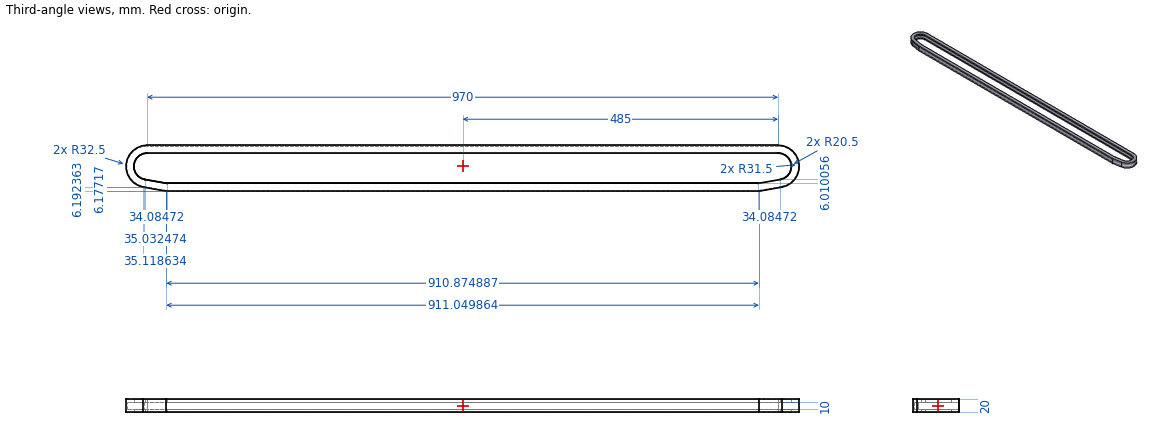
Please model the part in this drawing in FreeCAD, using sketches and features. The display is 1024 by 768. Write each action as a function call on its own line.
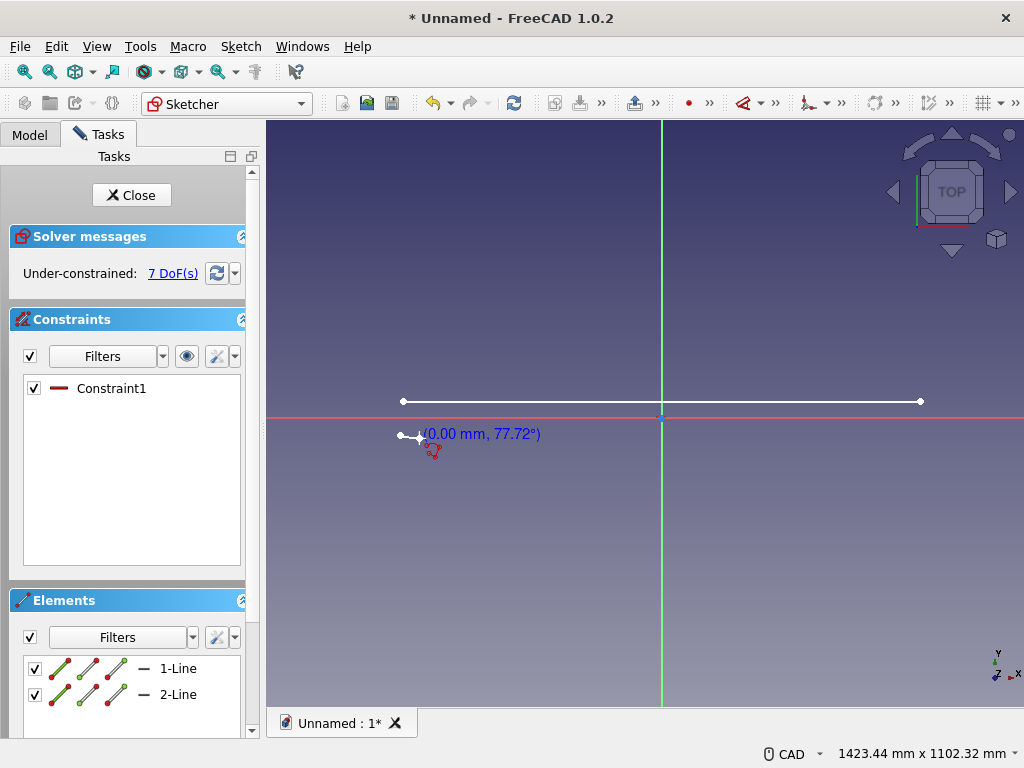
scroll(403, 401, down, 2)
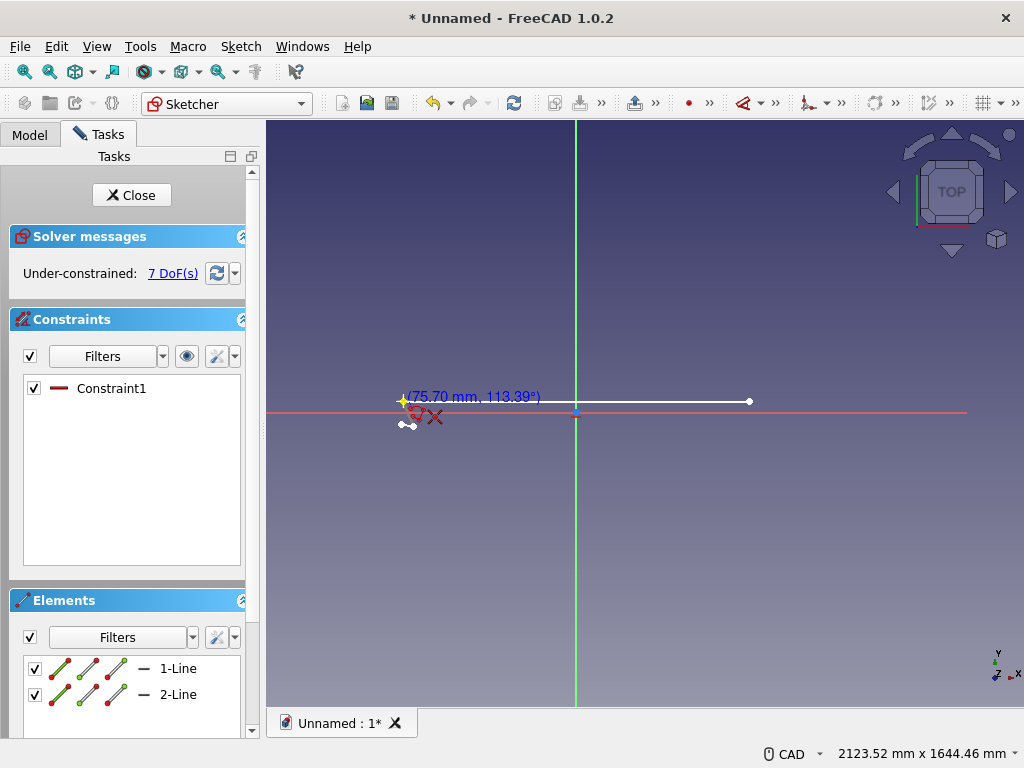
click(739, 426)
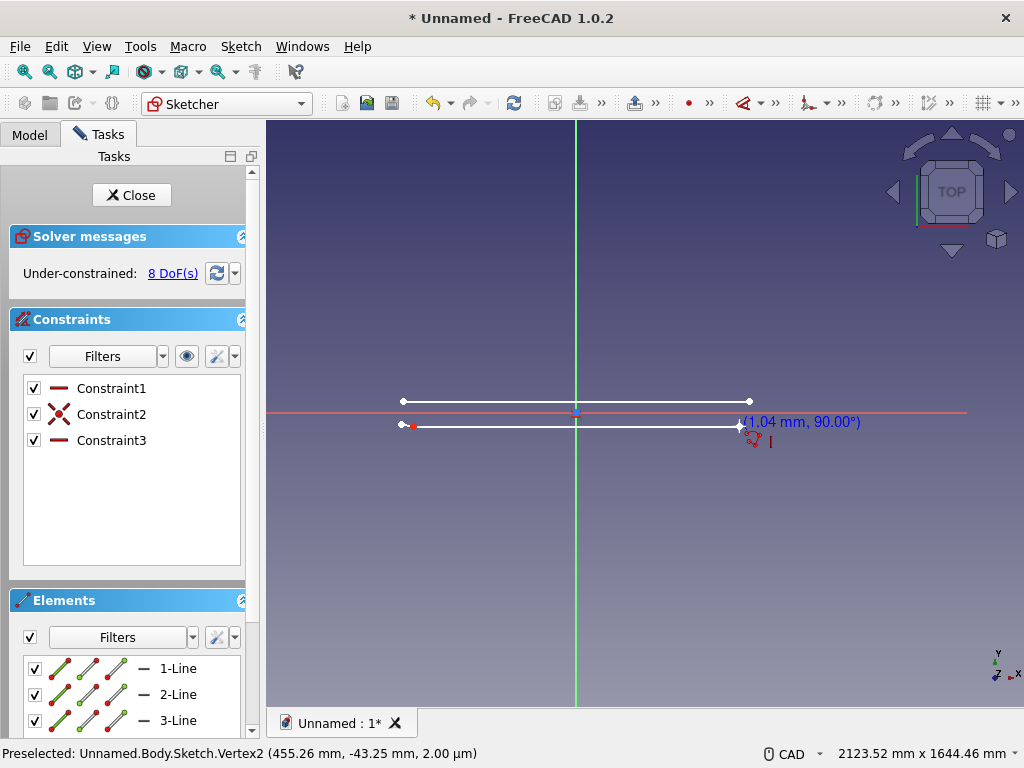
scroll(752, 424, up, 2)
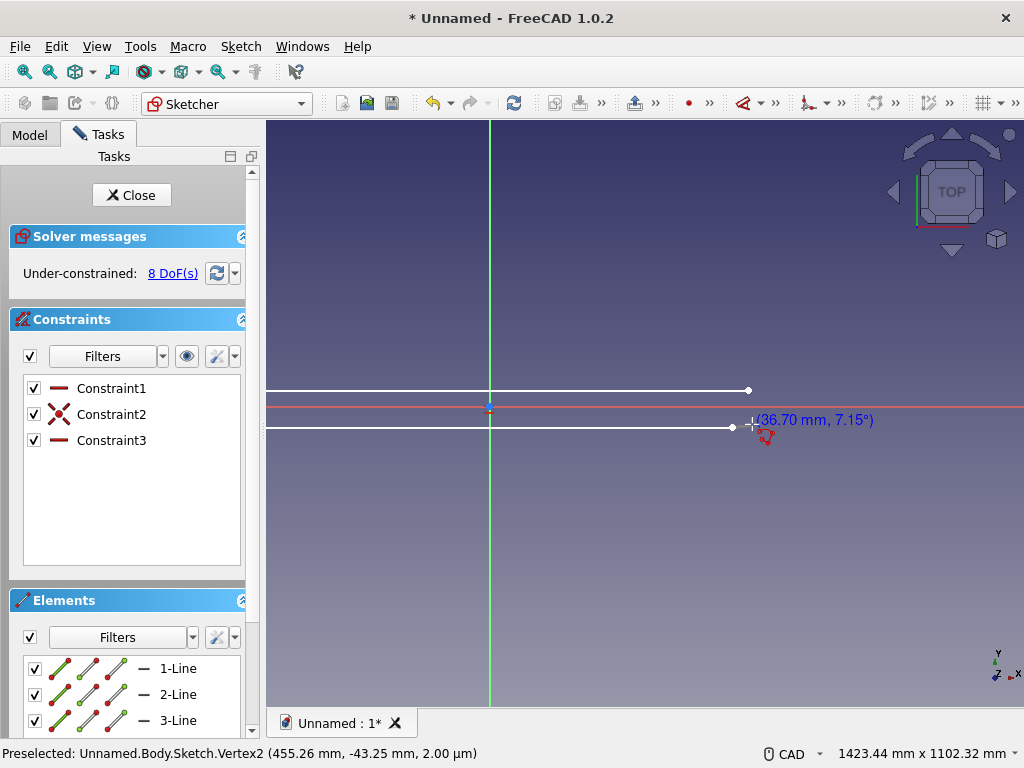
click(751, 424)
right_click(751, 424)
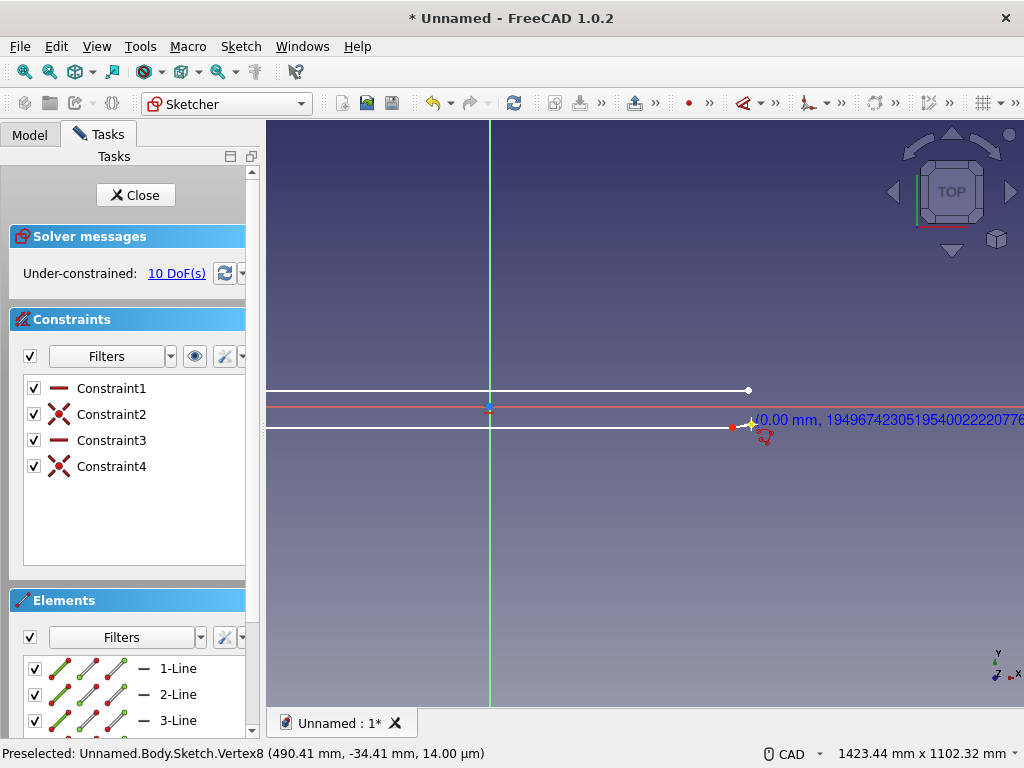
key(g)
key(3)
key(a)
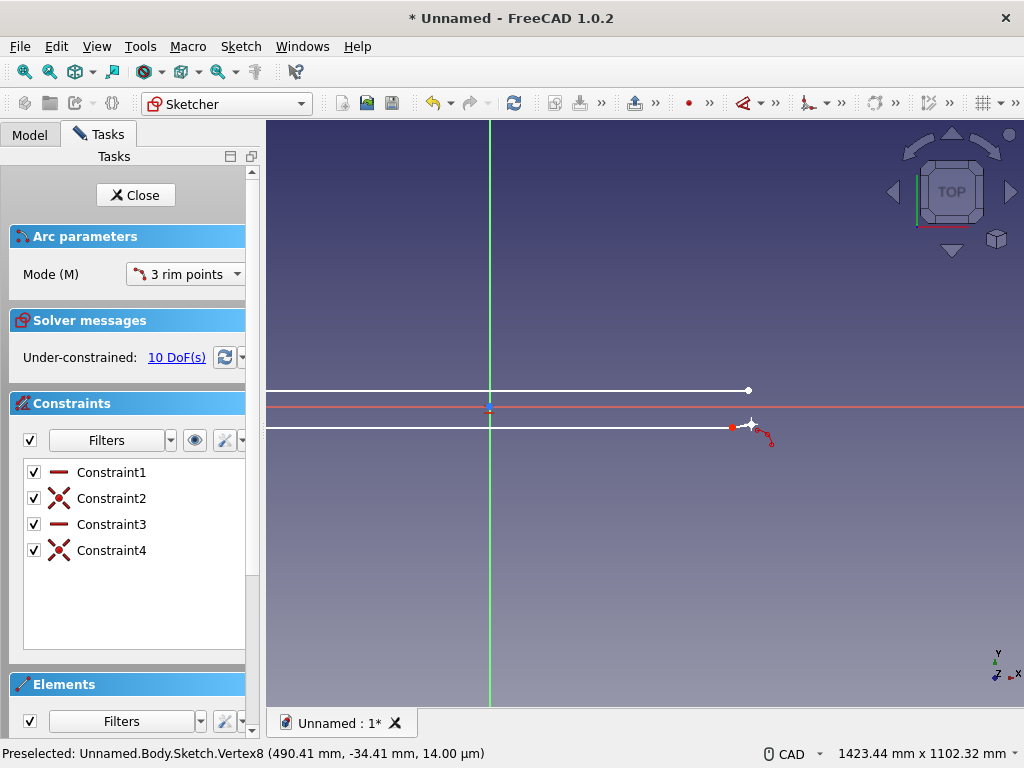
scroll(753, 424, down, 2)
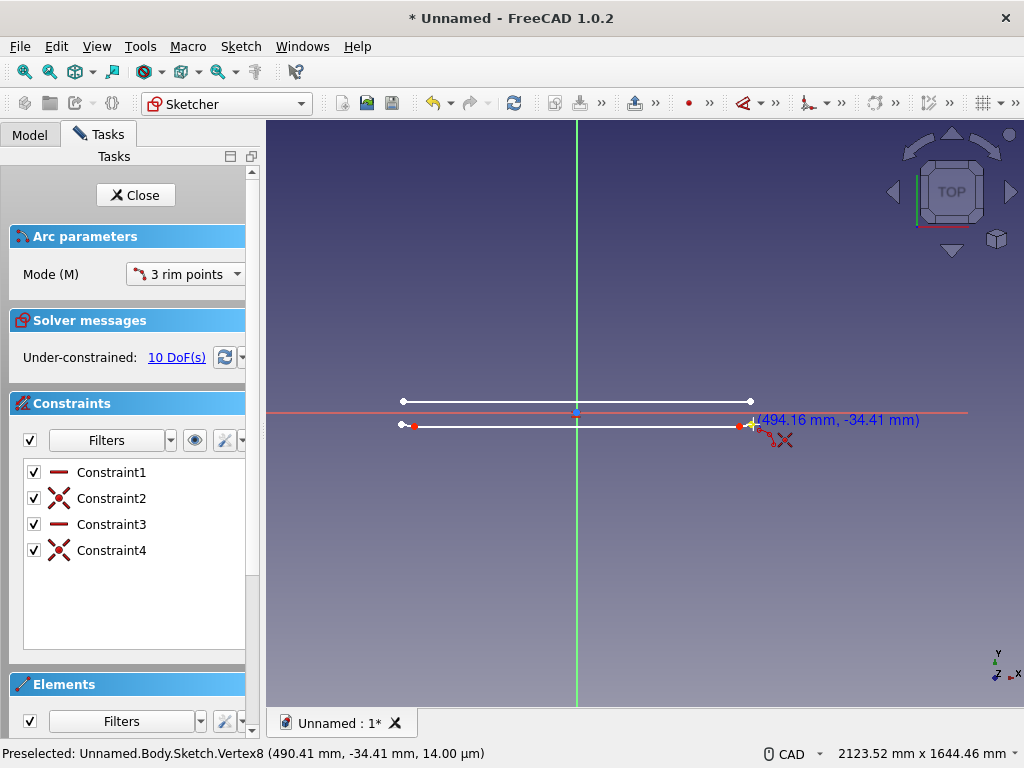
scroll(404, 401, up, 2)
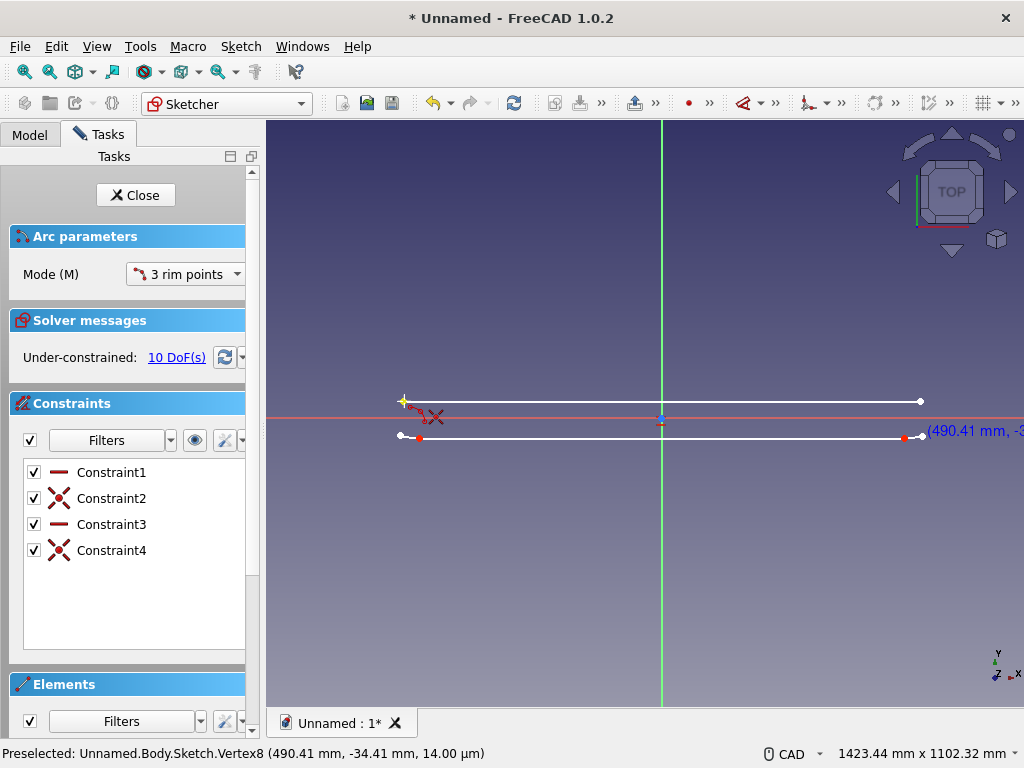
click(403, 402)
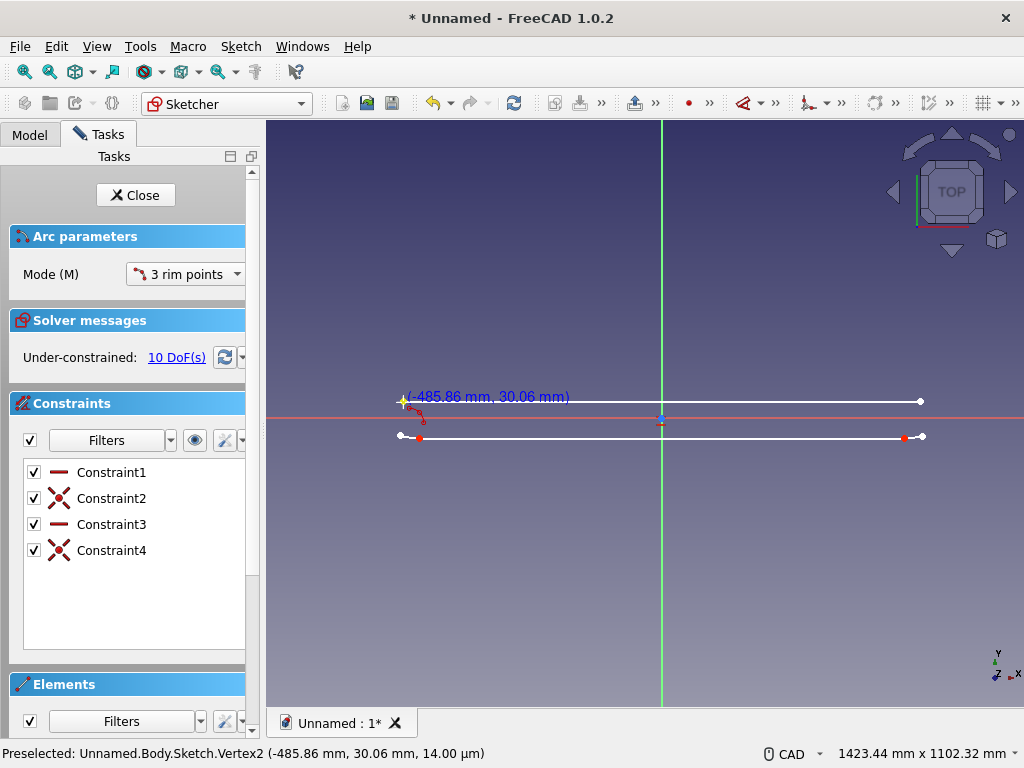
scroll(400, 435, up, 3)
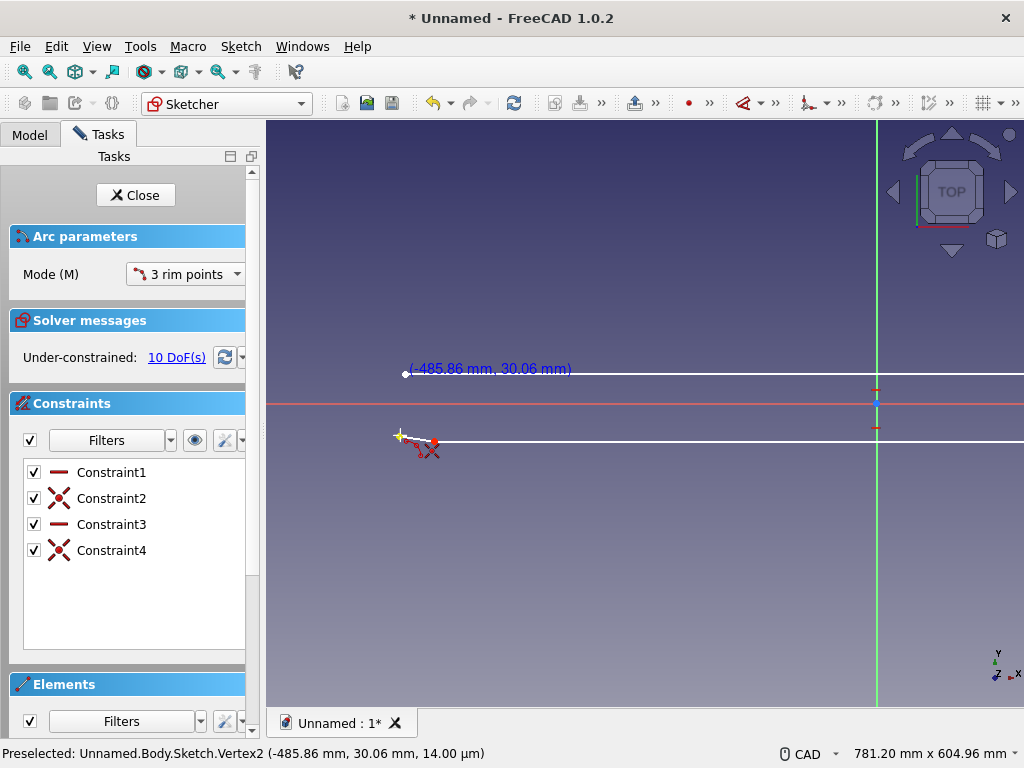
click(400, 436)
click(382, 384)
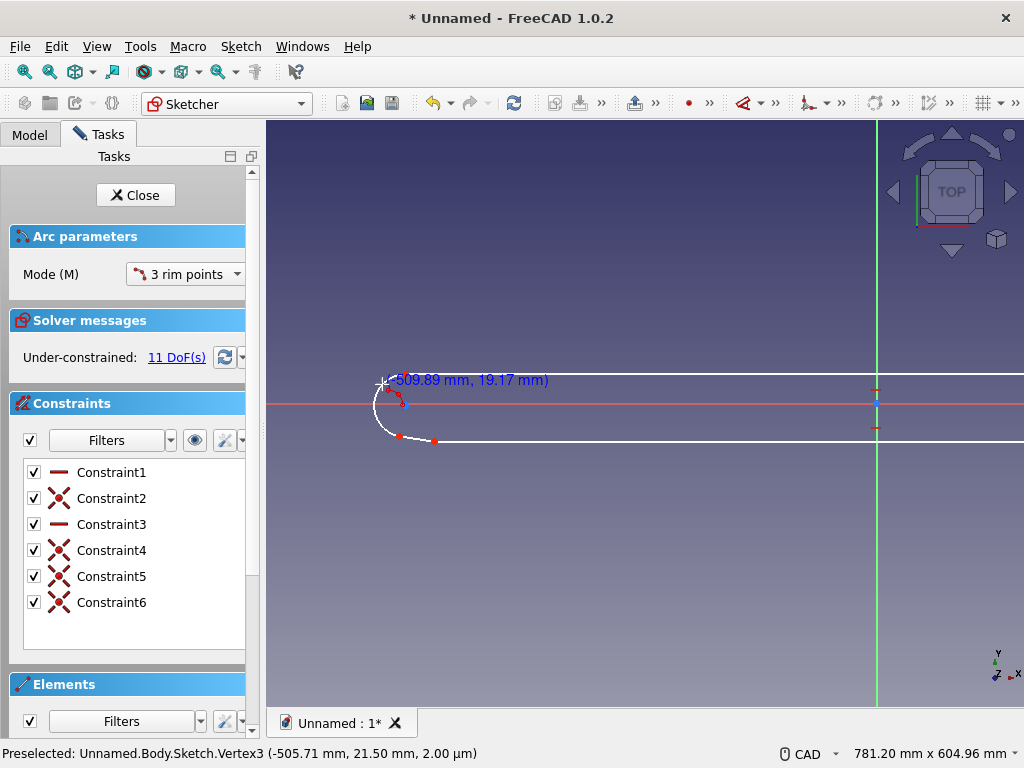
scroll(402, 418, down, 5)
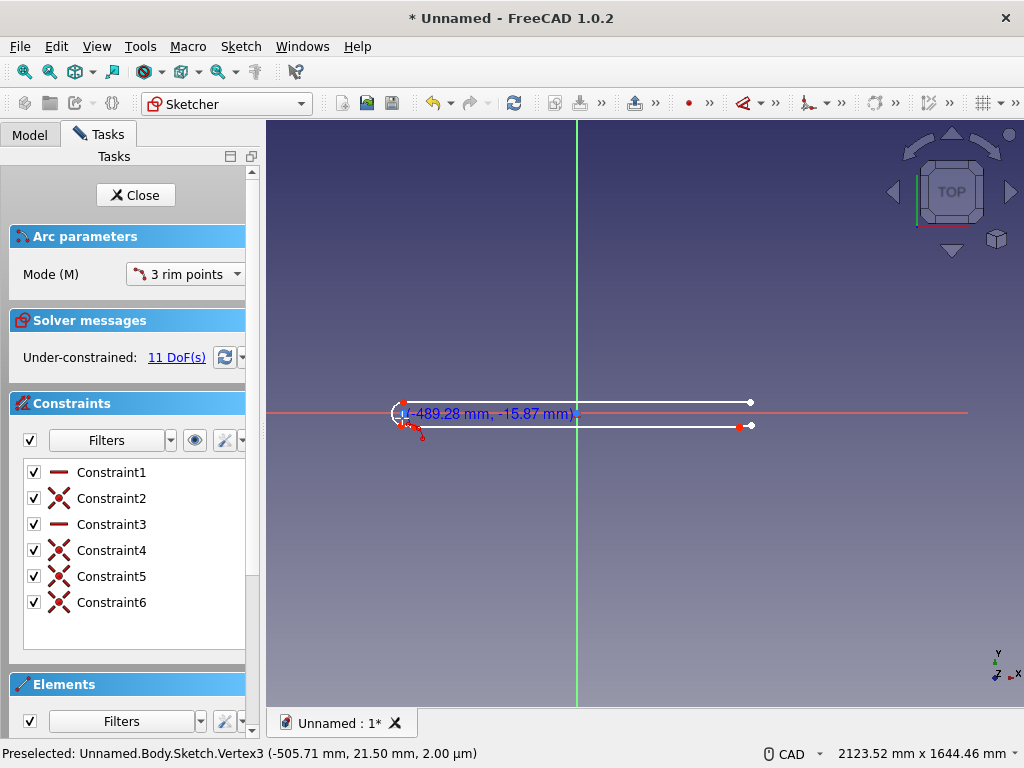
scroll(752, 424, up, 5)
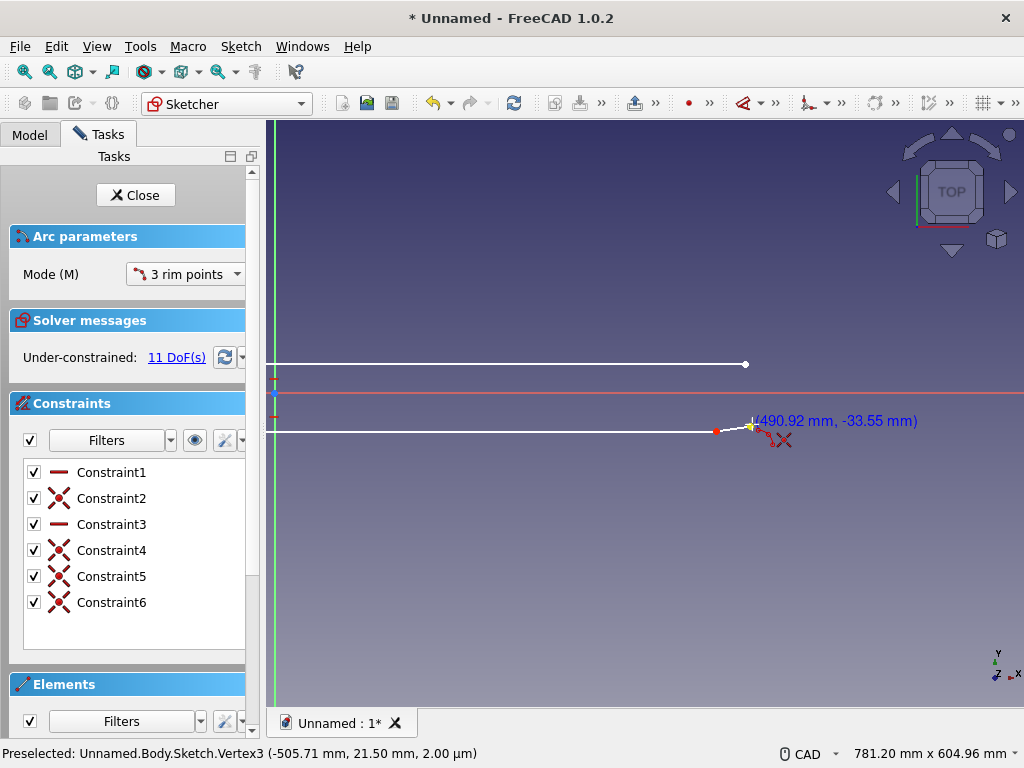
click(750, 427)
click(746, 364)
click(770, 373)